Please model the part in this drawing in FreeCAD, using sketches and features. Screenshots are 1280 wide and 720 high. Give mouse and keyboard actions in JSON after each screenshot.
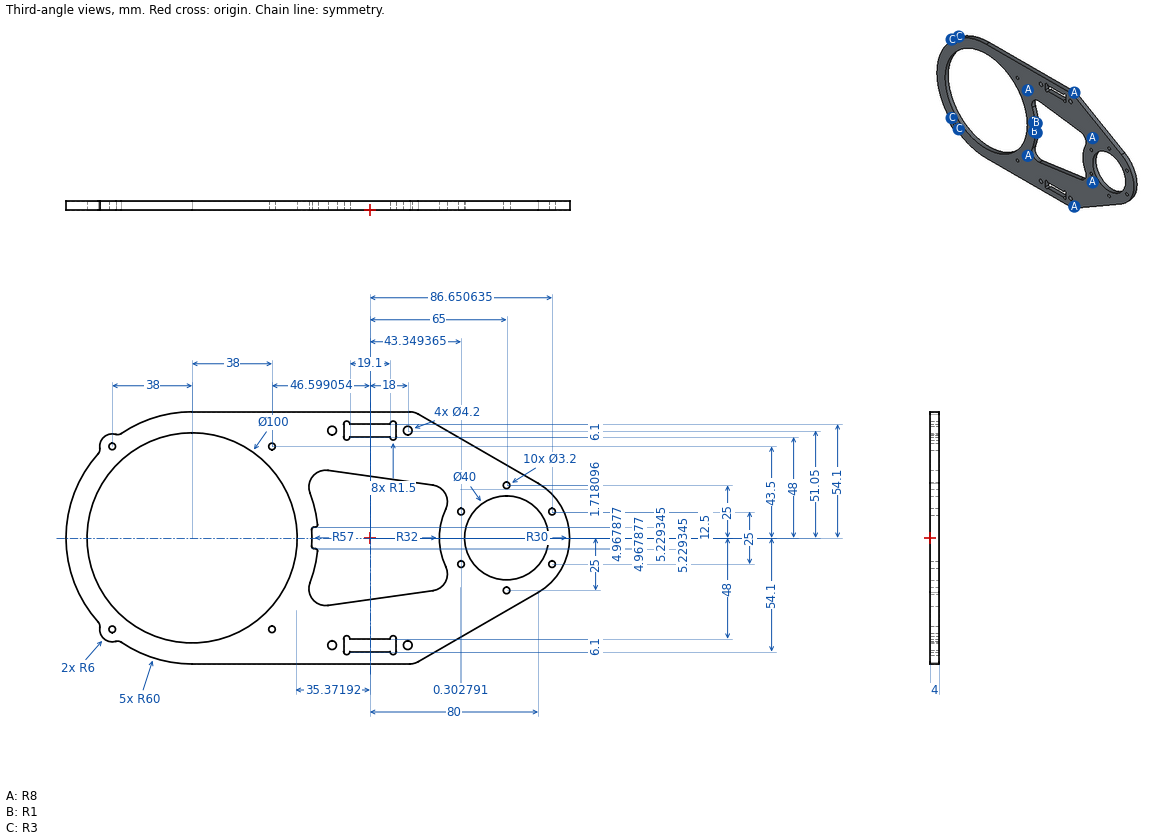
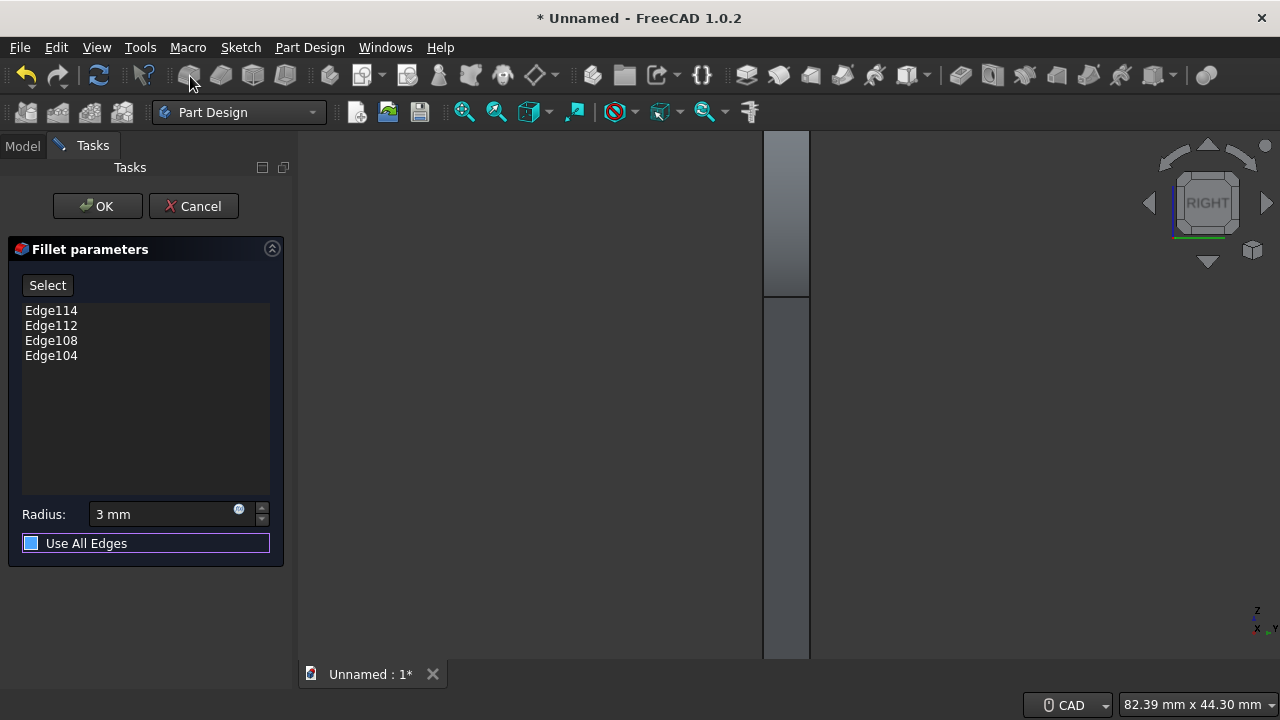
{"action": "left_click", "coordinate": [98, 206]}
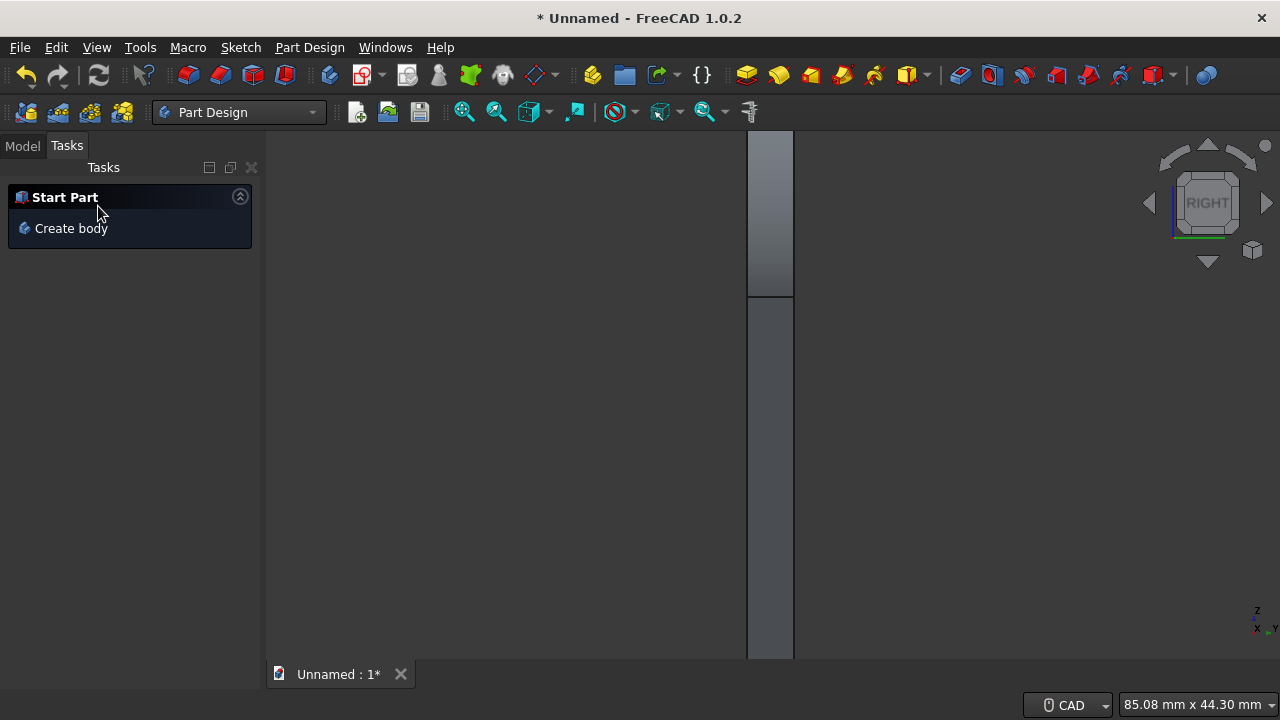
{"action": "key", "text": "0"}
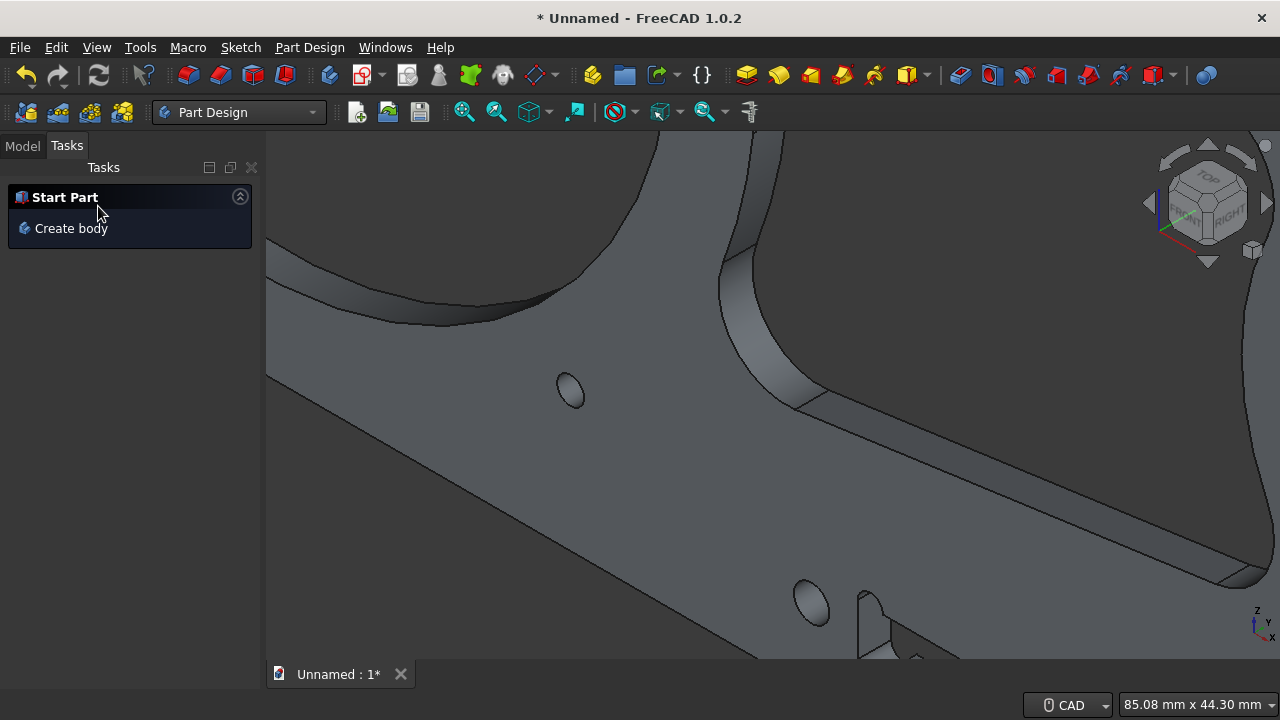
{"action": "left_click", "coordinate": [466, 112]}